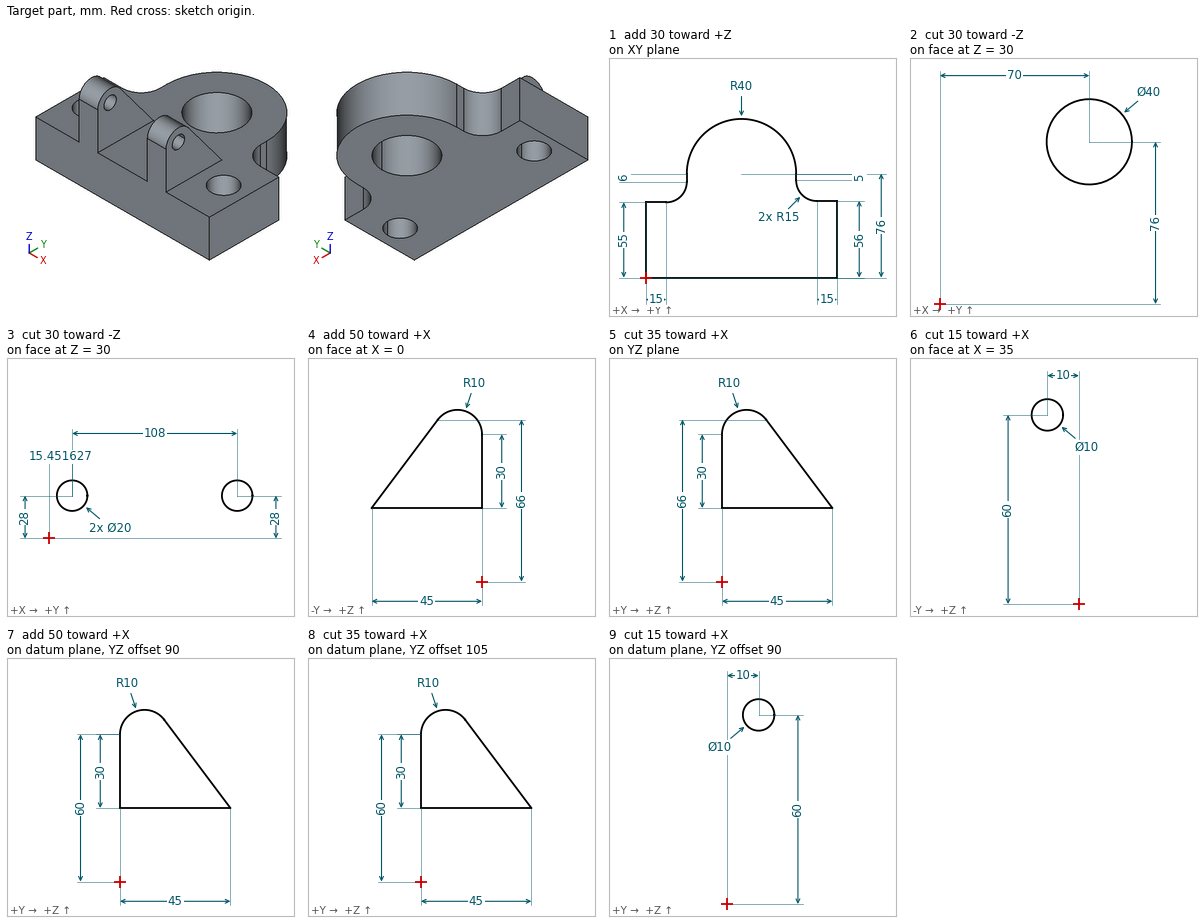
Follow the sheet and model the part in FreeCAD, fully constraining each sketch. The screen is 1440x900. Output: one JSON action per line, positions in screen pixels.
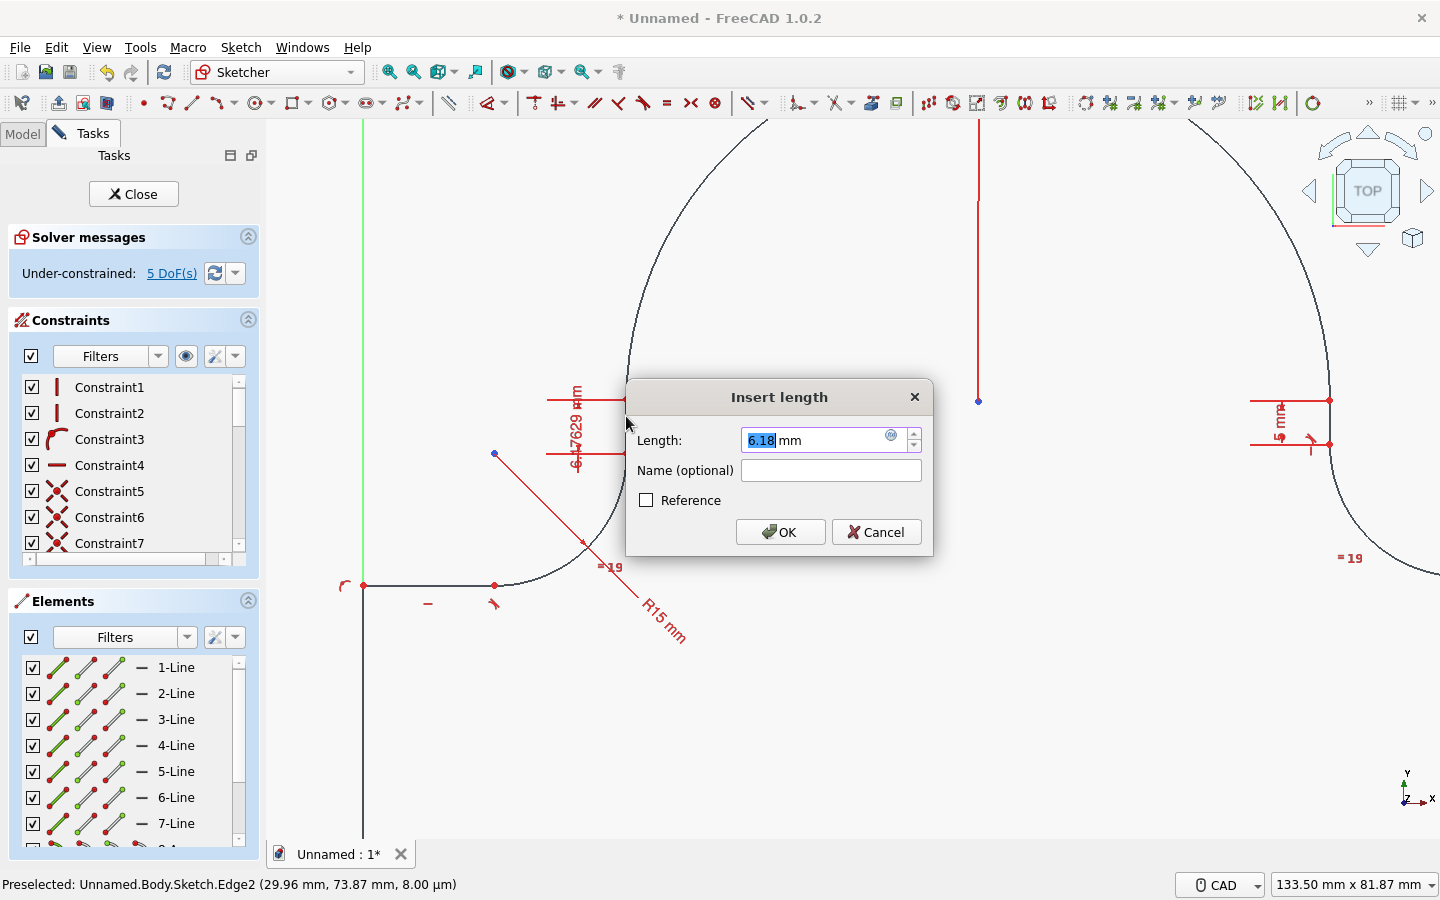
{"action": "type", "text": "6"}
{"action": "key", "text": "Return"}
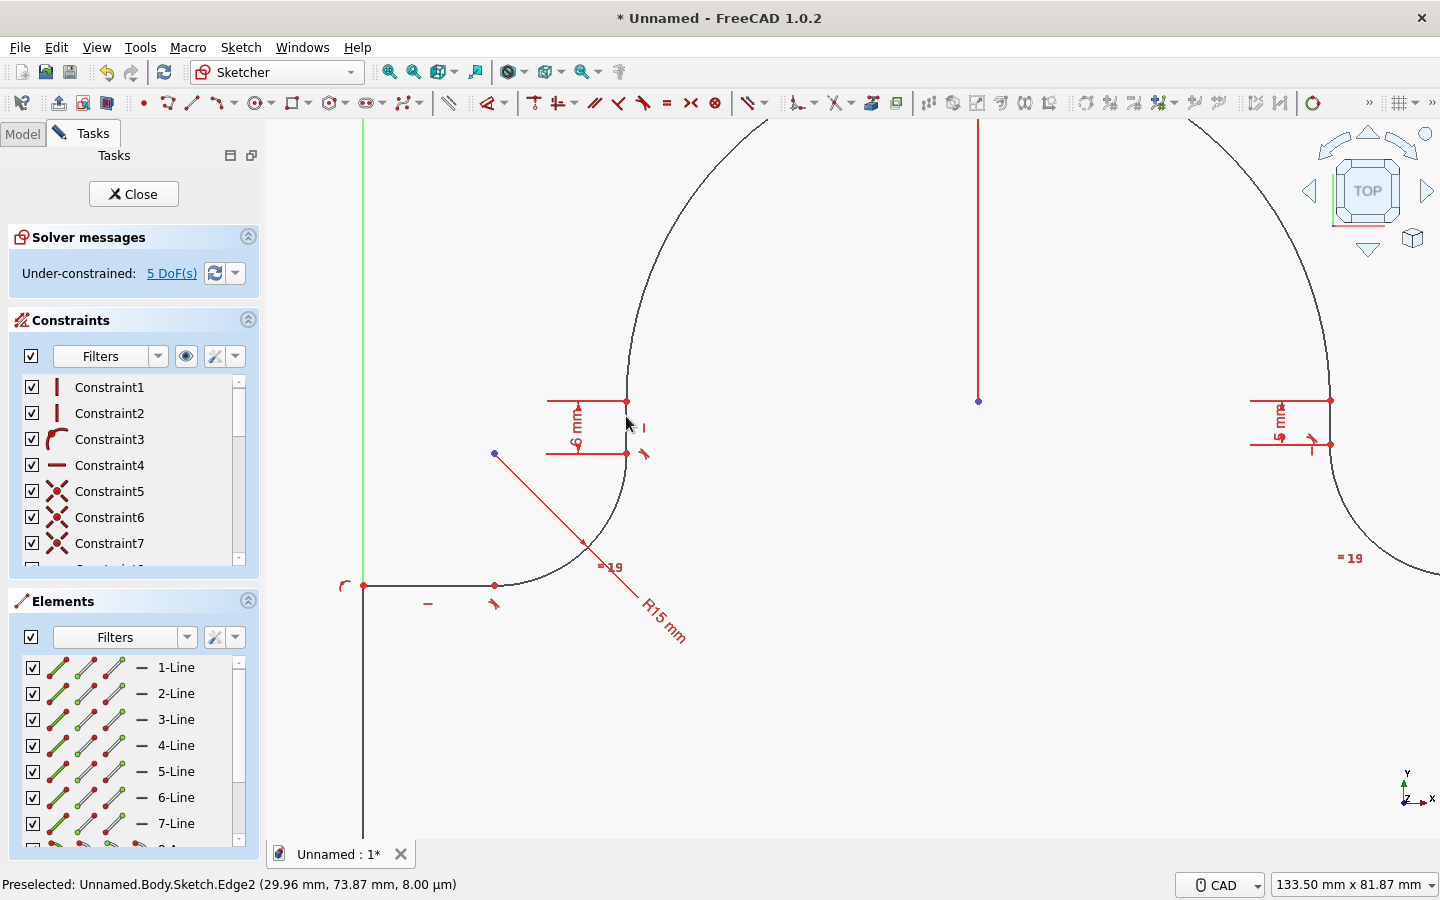
{"action": "left_click", "coordinate": [455, 586]}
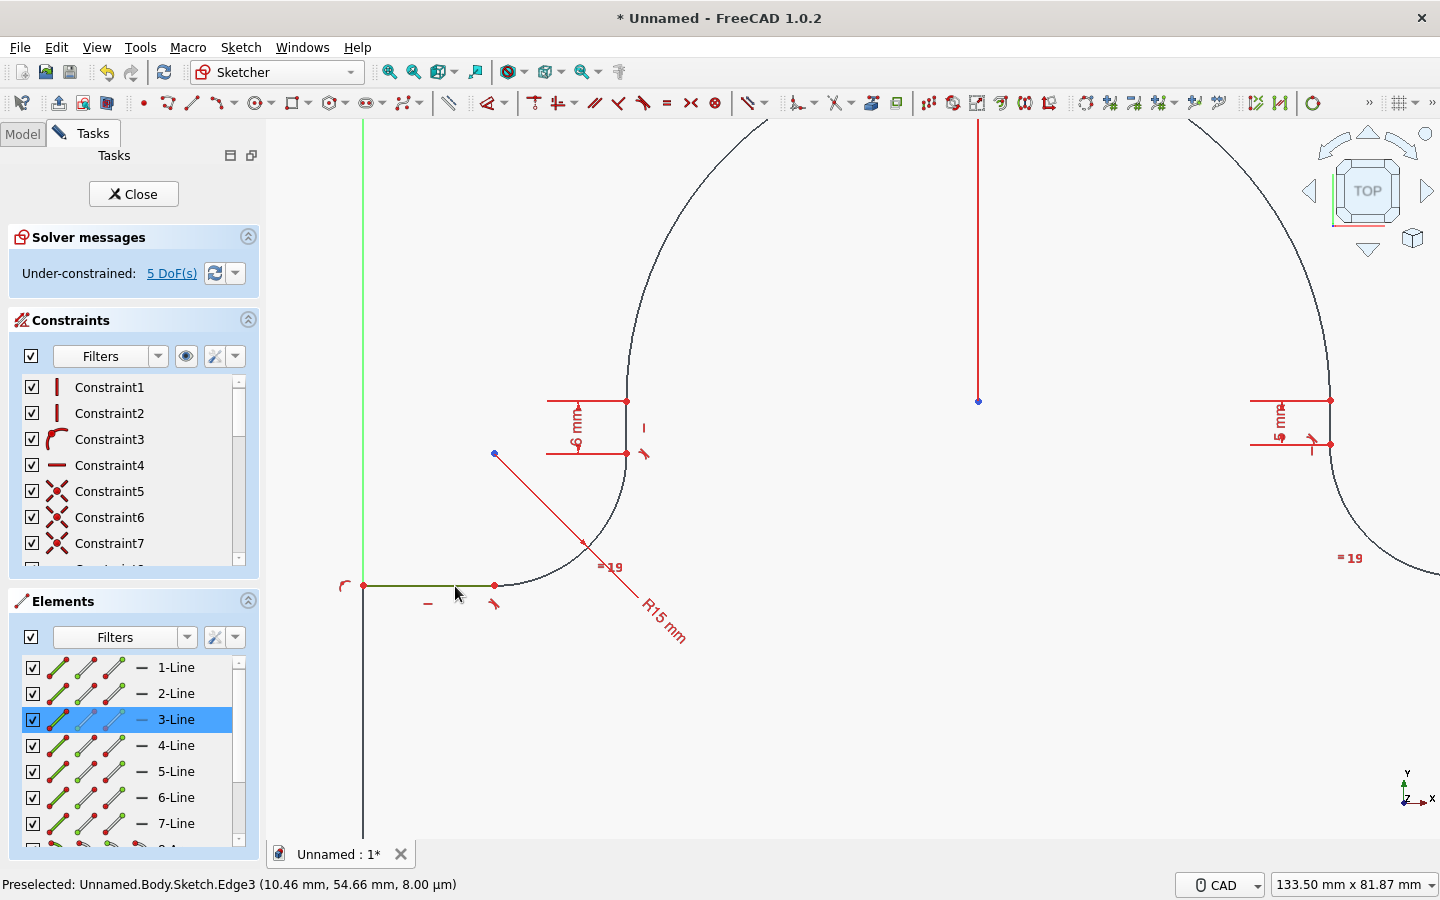
{"action": "key", "text": "l"}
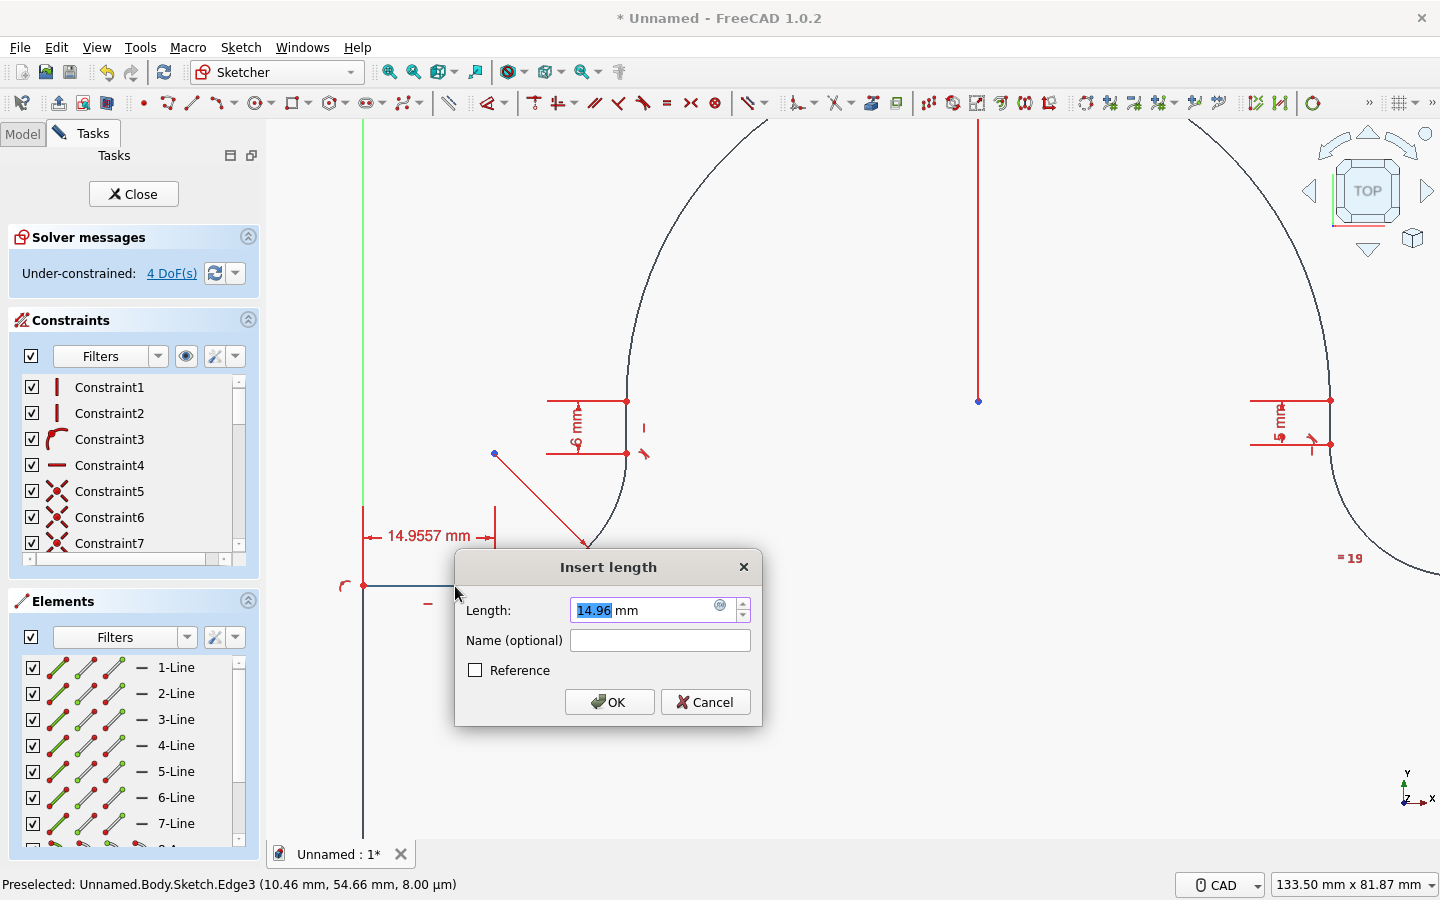
{"action": "type", "text": "15"}
{"action": "key", "text": "Return"}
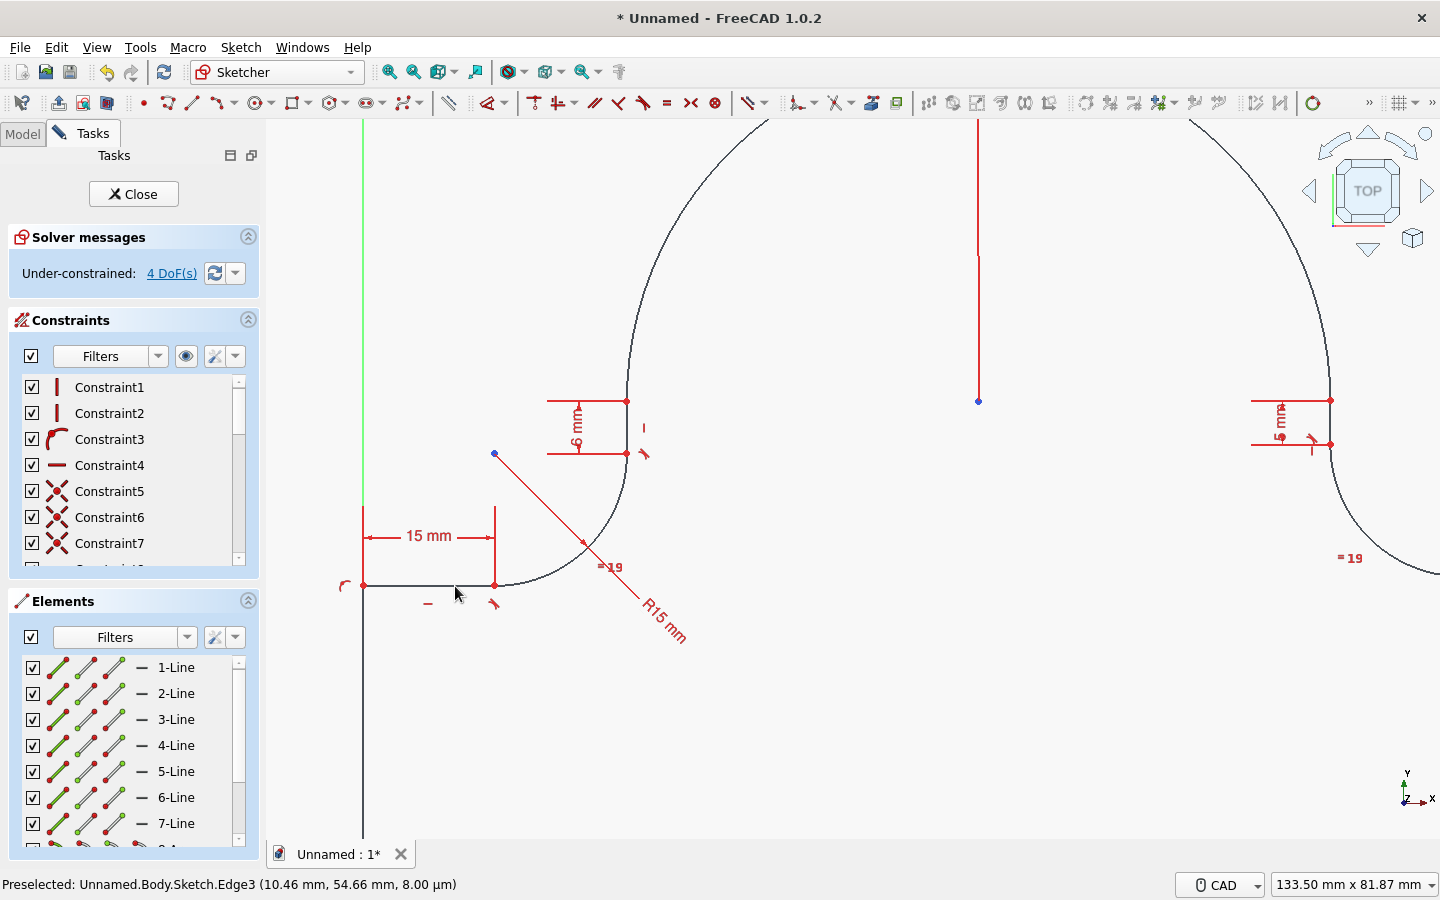
{"action": "left_click", "coordinate": [363, 730]}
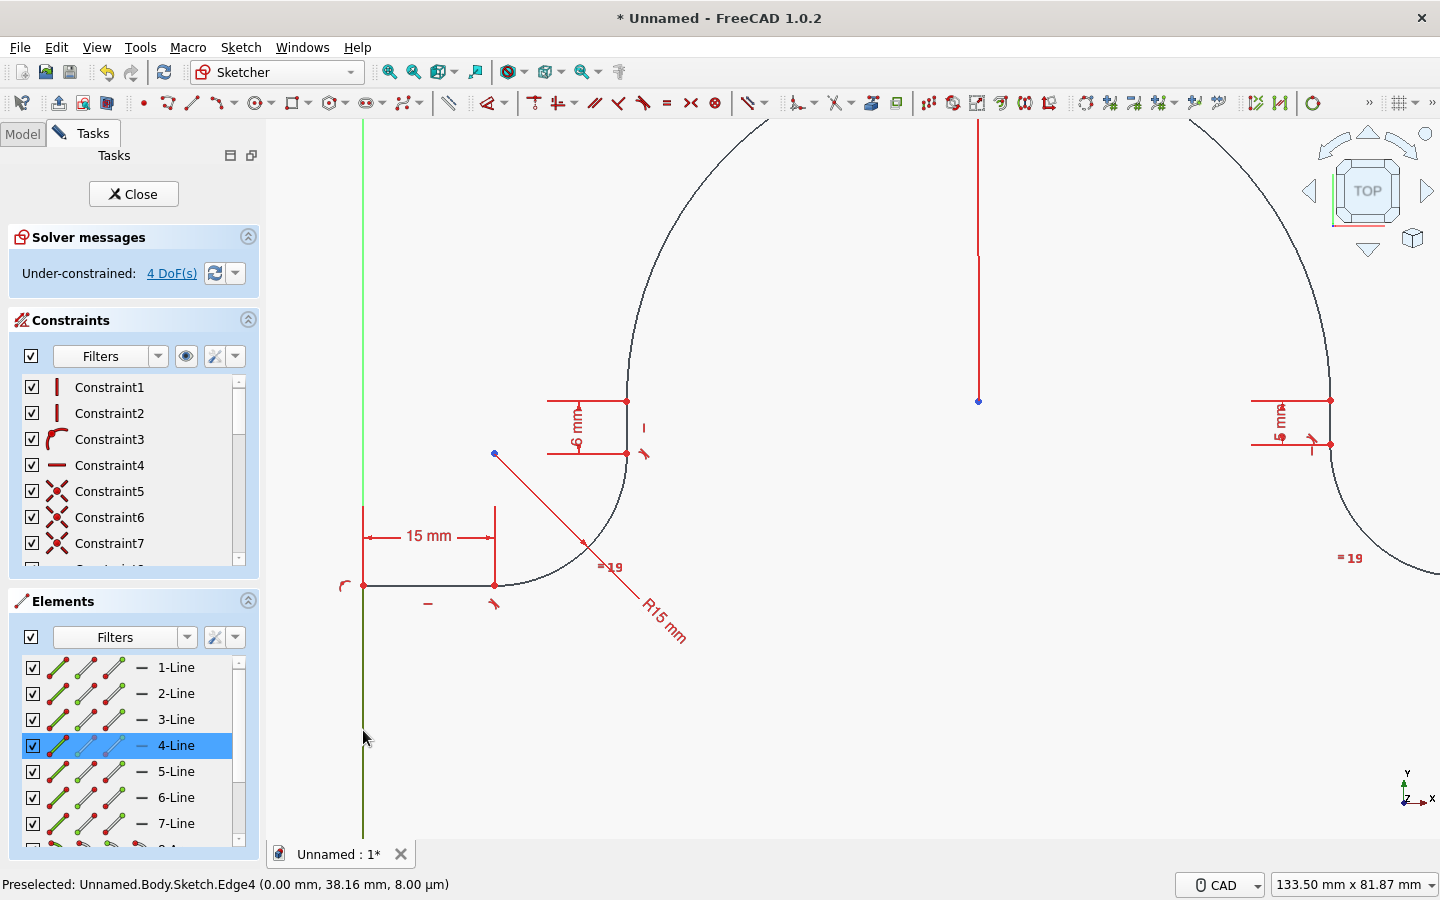
{"action": "key", "text": "i"}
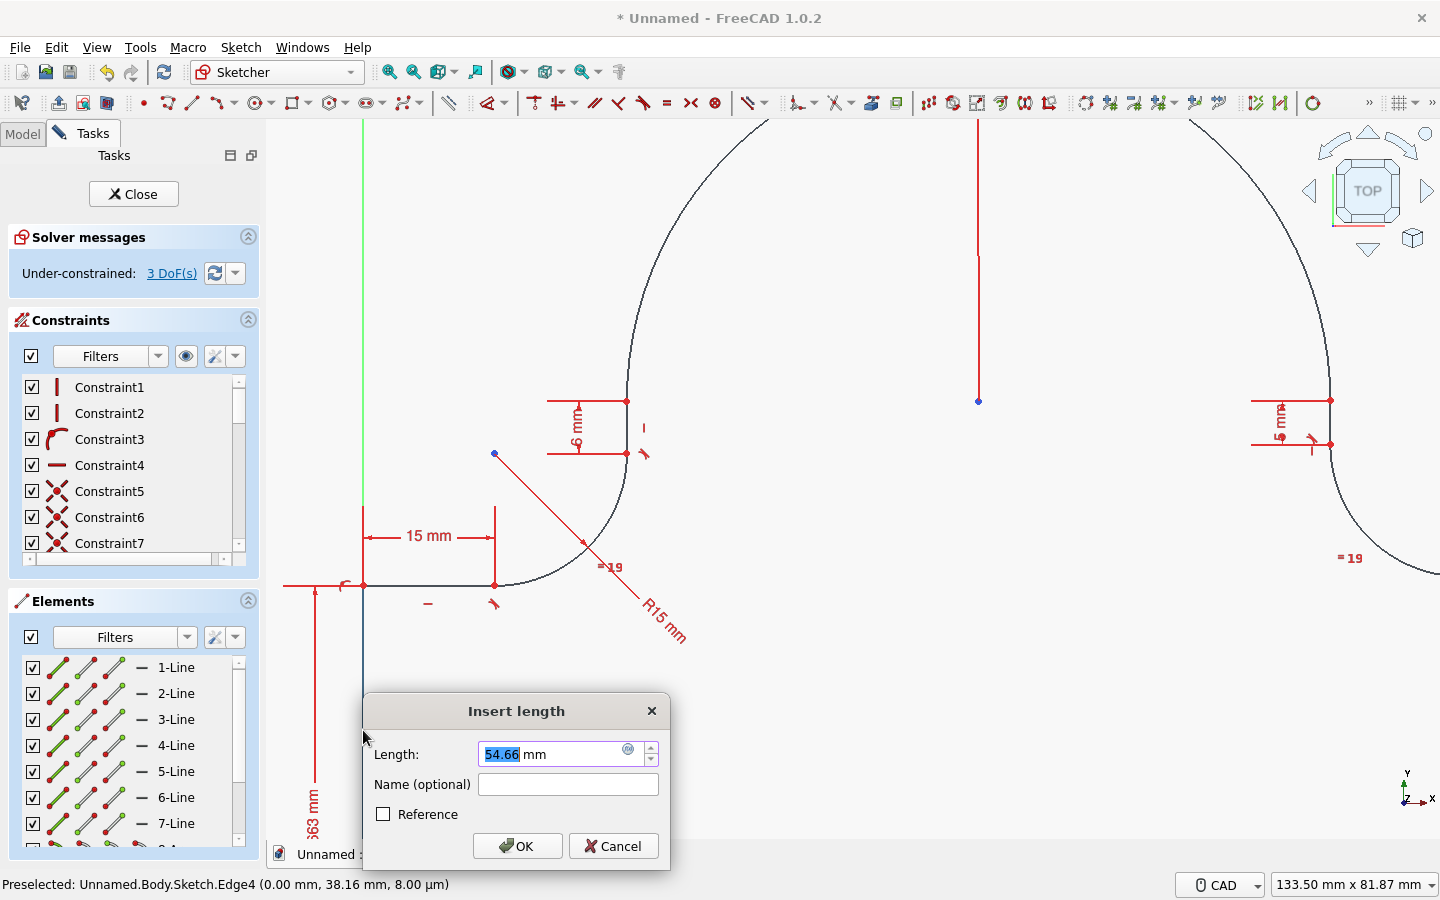
{"action": "type", "text": "55"}
{"action": "key", "text": "Return"}